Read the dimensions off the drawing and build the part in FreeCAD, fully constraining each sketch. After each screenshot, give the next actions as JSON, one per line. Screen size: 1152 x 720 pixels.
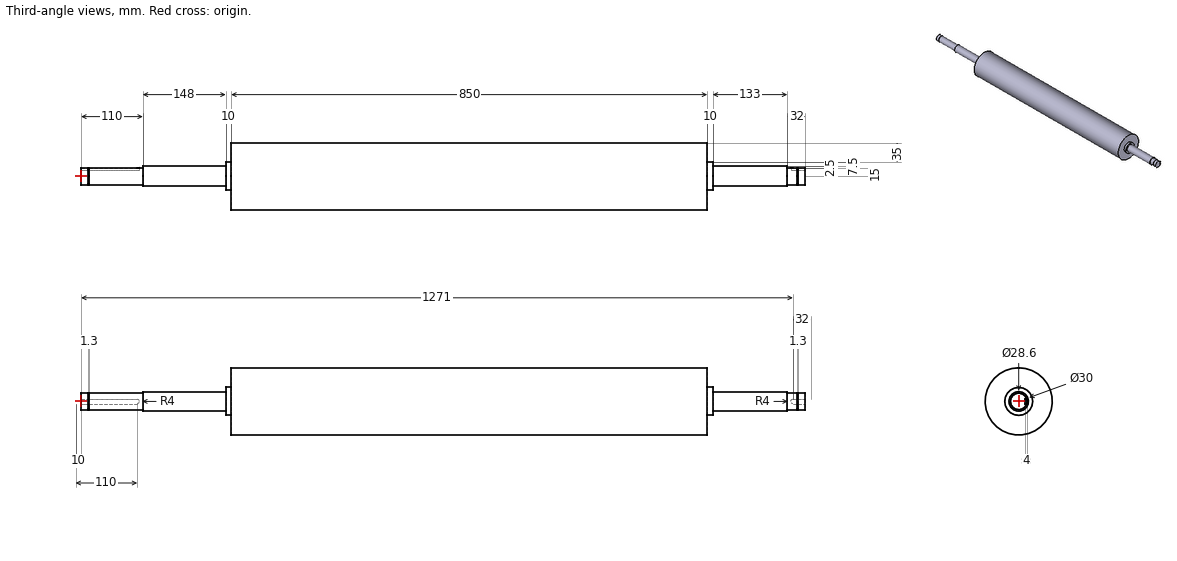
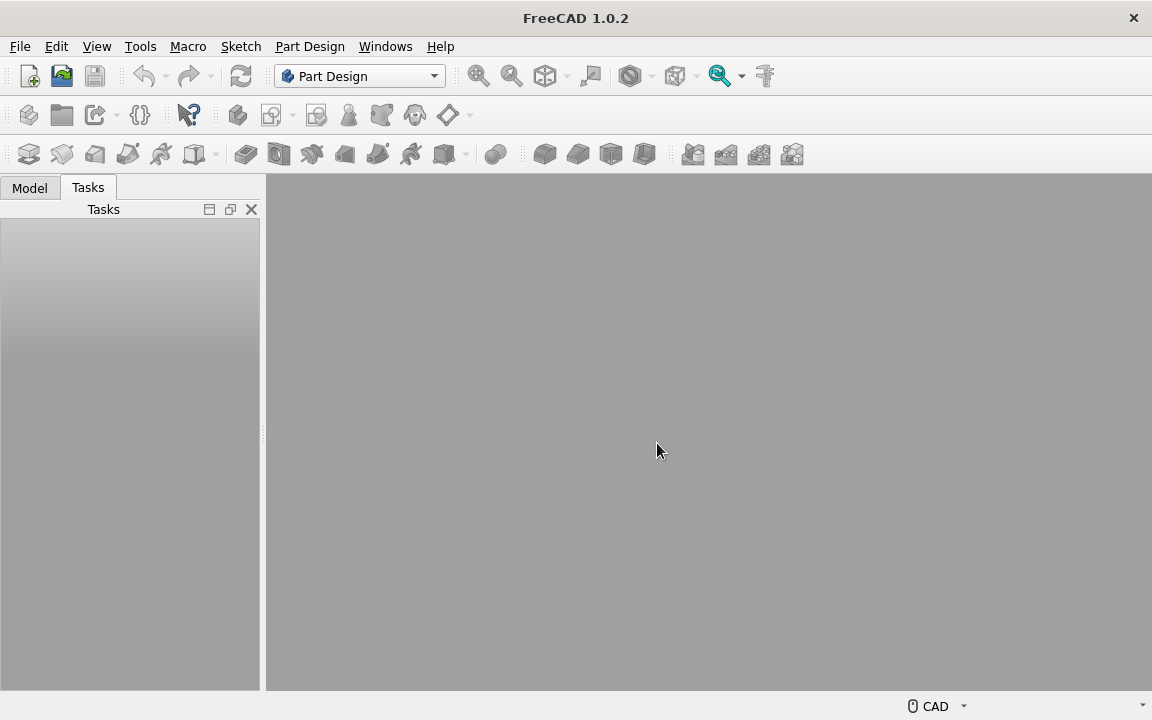
{"action": "key", "text": "ctrl+n"}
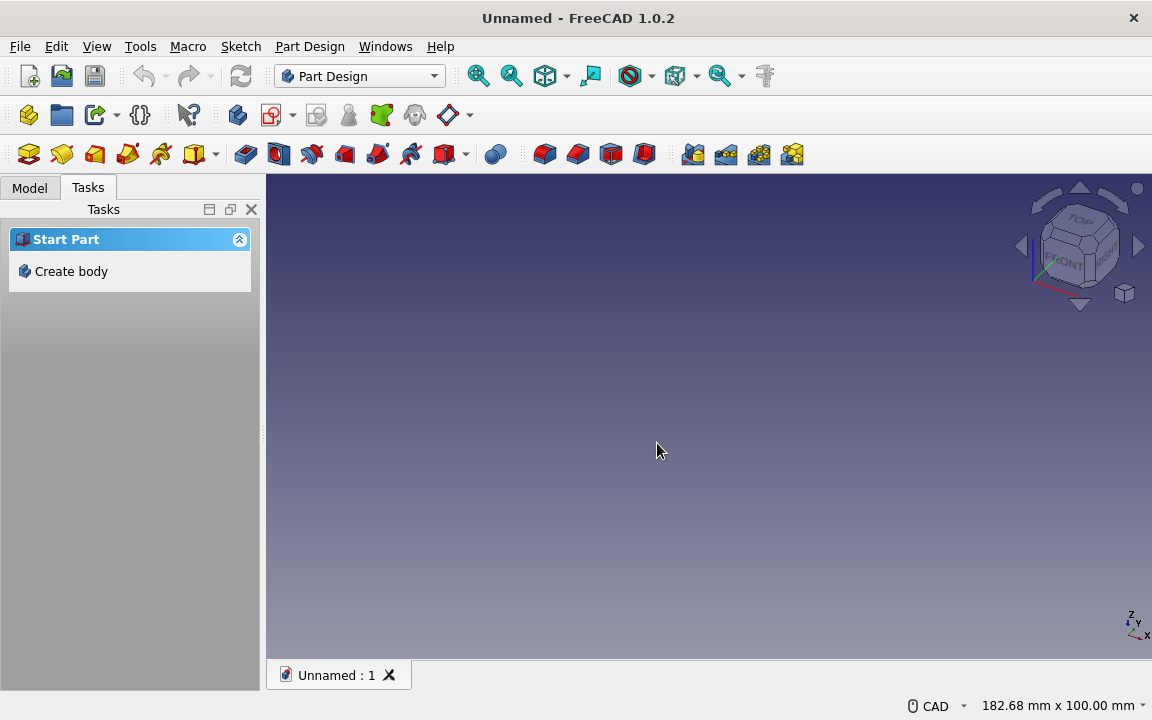
{"action": "left_click", "coordinate": [270, 116]}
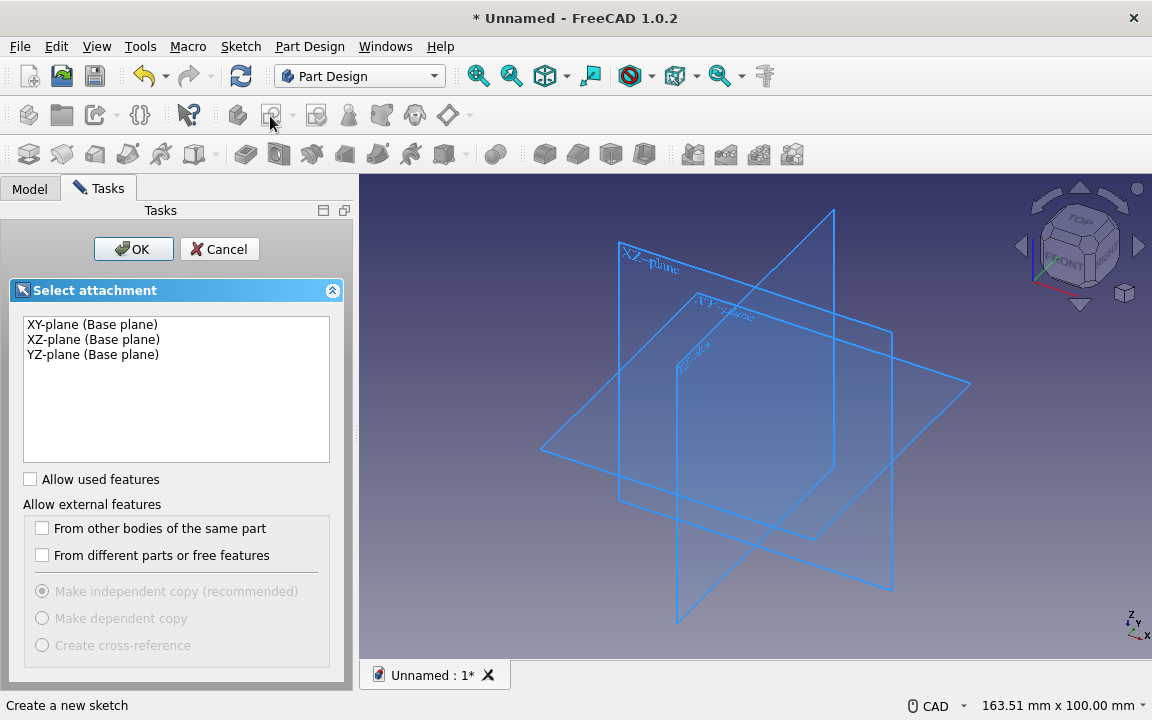
{"action": "left_click", "coordinate": [84, 324]}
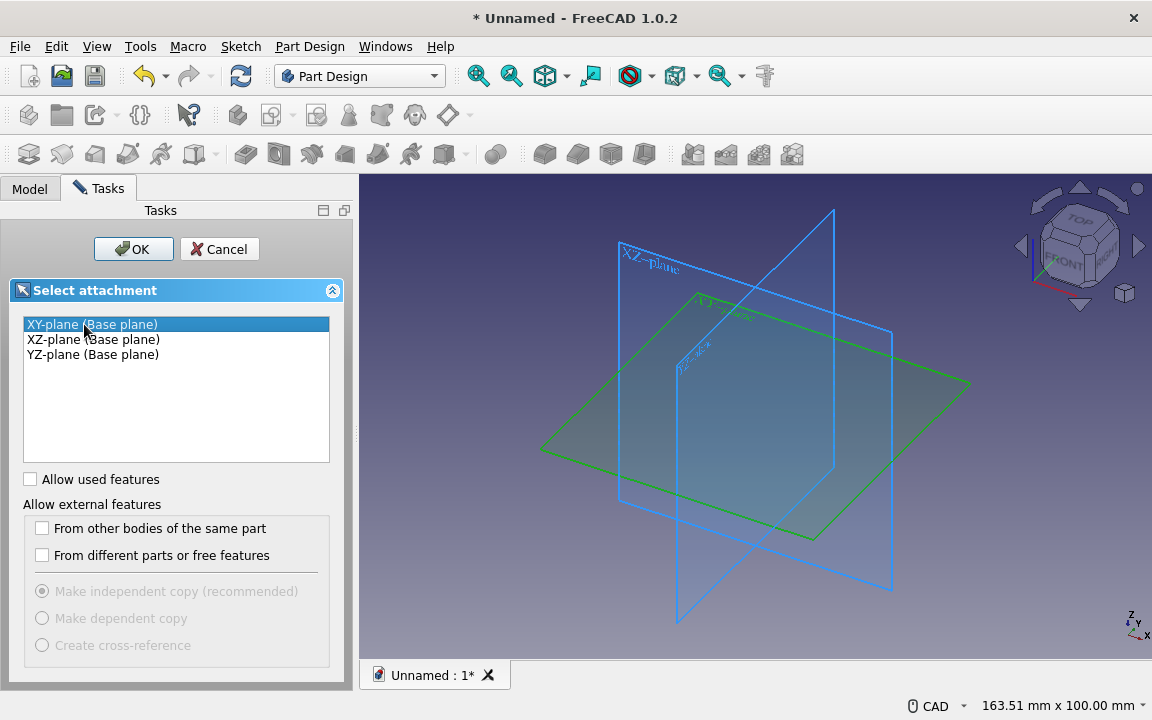
{"action": "left_click", "coordinate": [134, 249]}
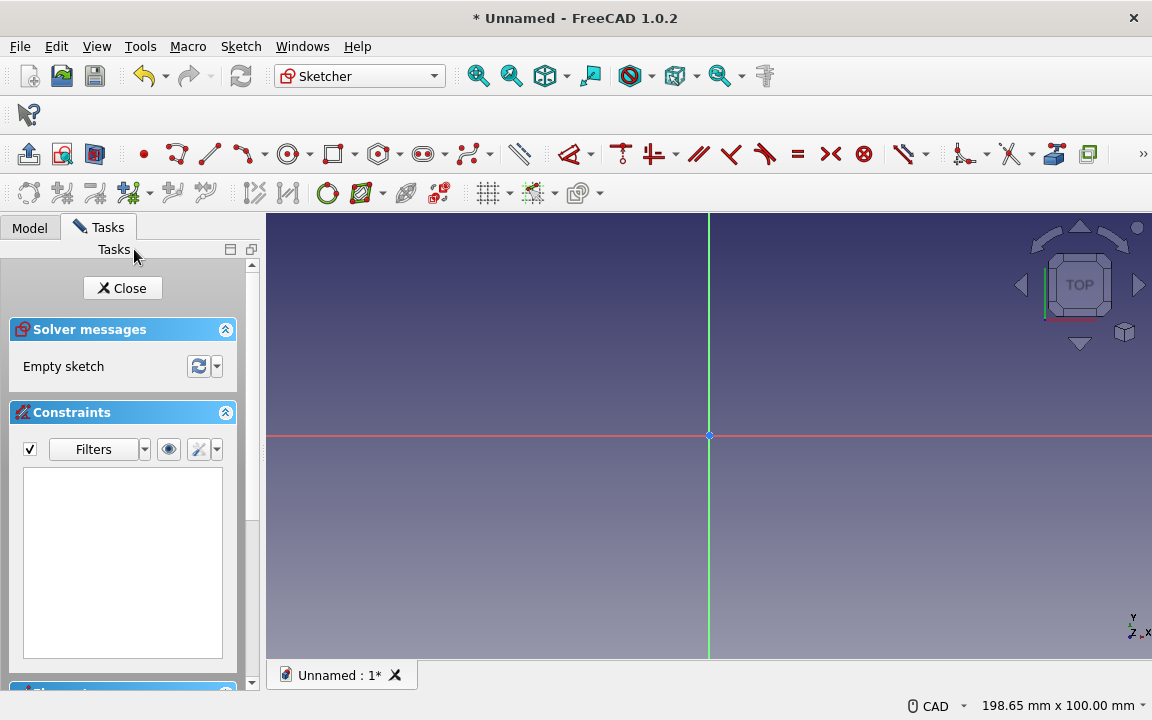
{"action": "scroll", "coordinate": [346, 449], "scroll_direction": "down", "scroll_amount": 12}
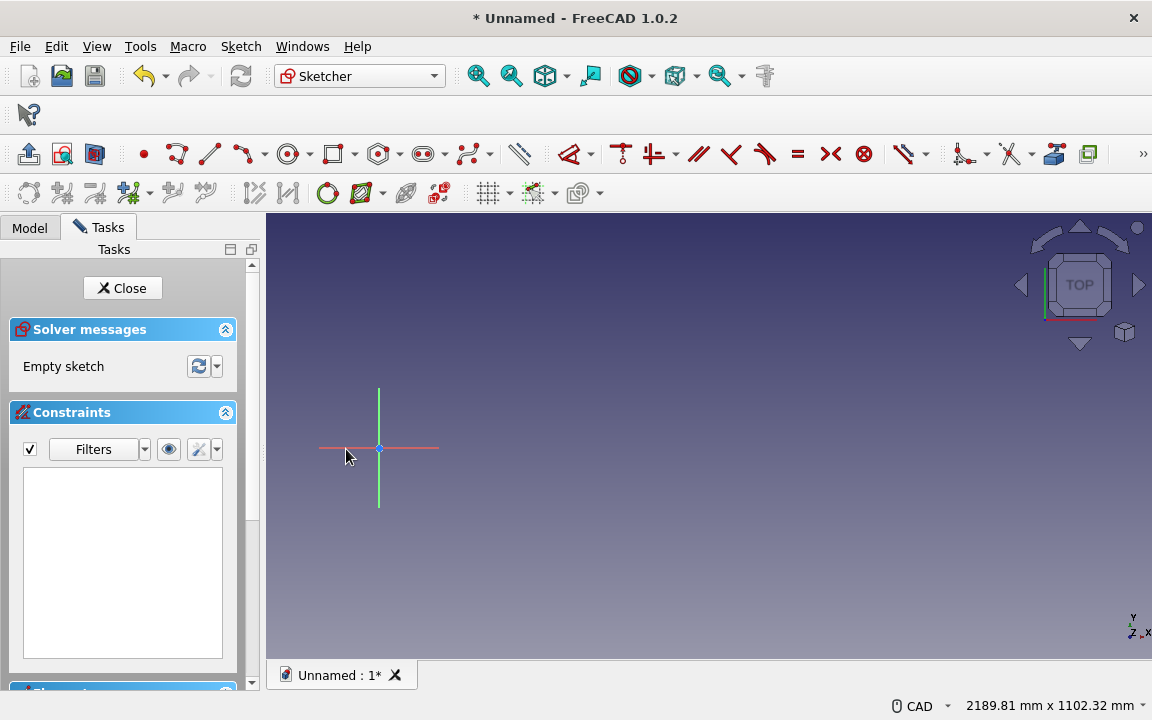
{"action": "left_click", "coordinate": [177, 154]}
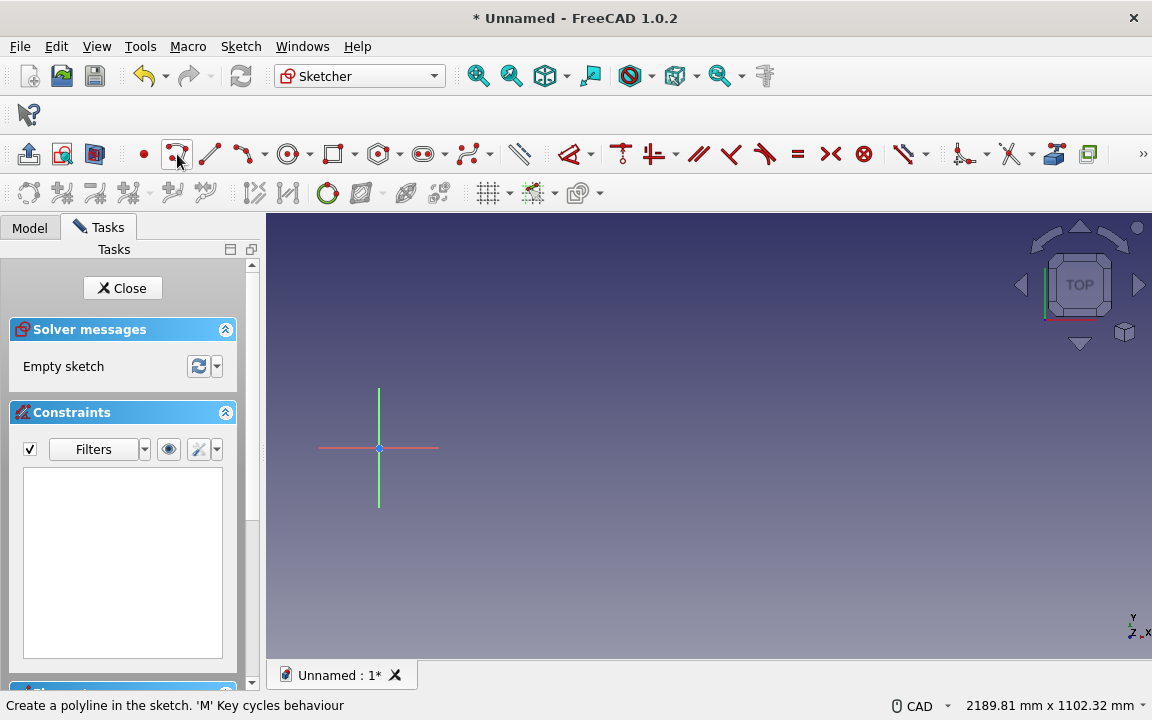
{"action": "left_click", "coordinate": [379, 448]}
{"action": "left_click", "coordinate": [902, 439]}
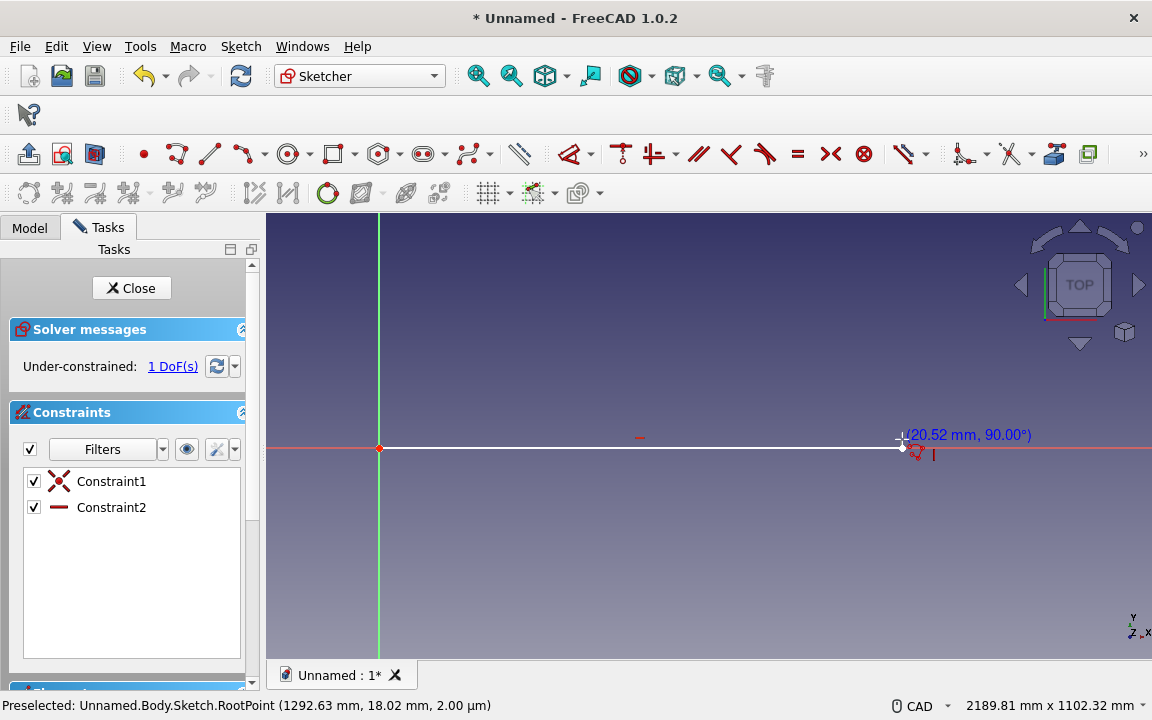
{"action": "scroll", "coordinate": [902, 442], "scroll_direction": "up", "scroll_amount": 5}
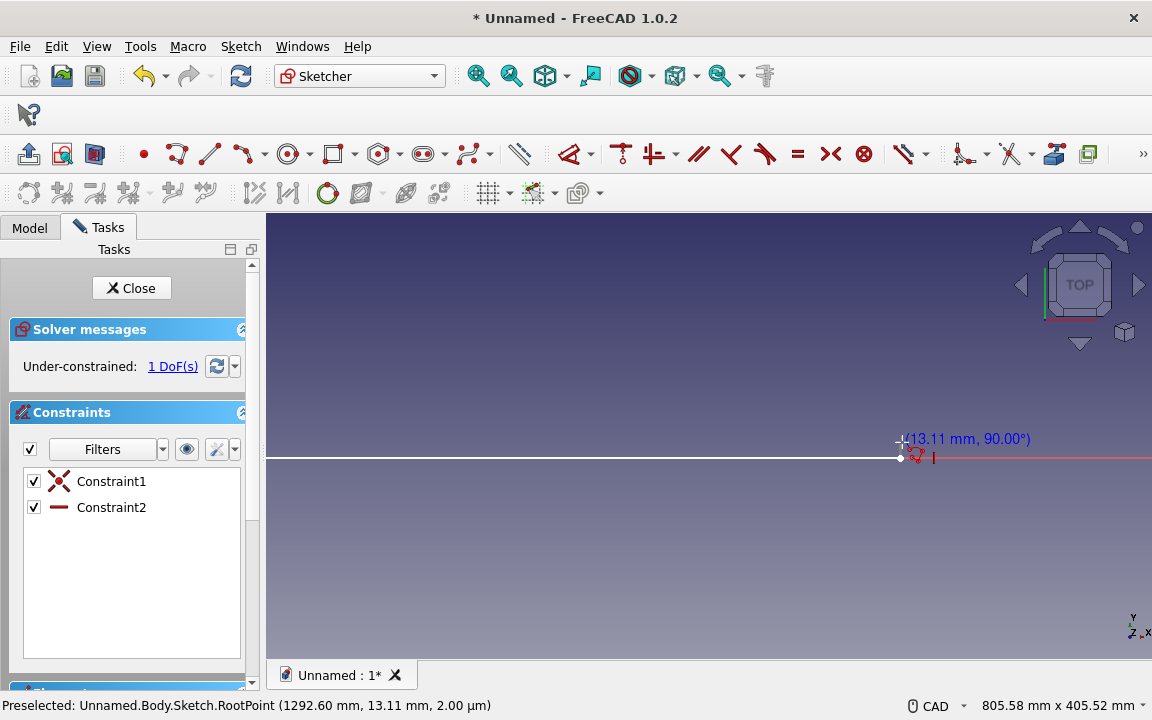
{"action": "left_click", "coordinate": [901, 442]}
{"action": "left_click", "coordinate": [866, 442]}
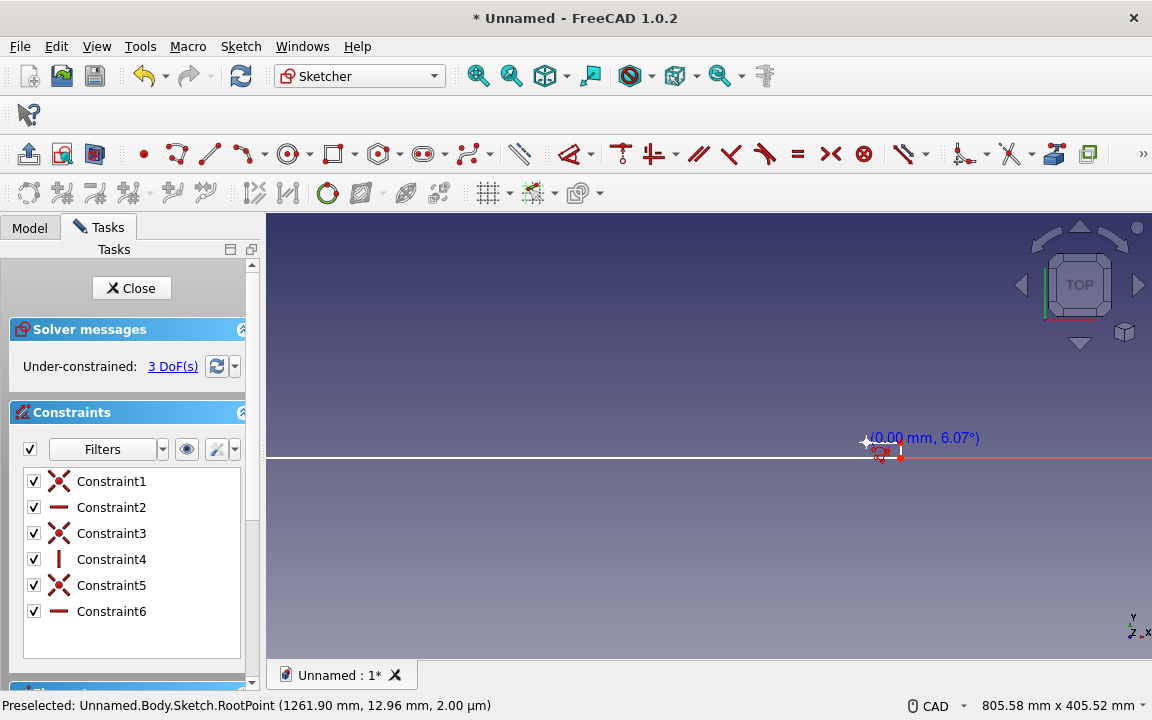
{"action": "scroll", "coordinate": [866, 439], "scroll_direction": "up", "scroll_amount": 9}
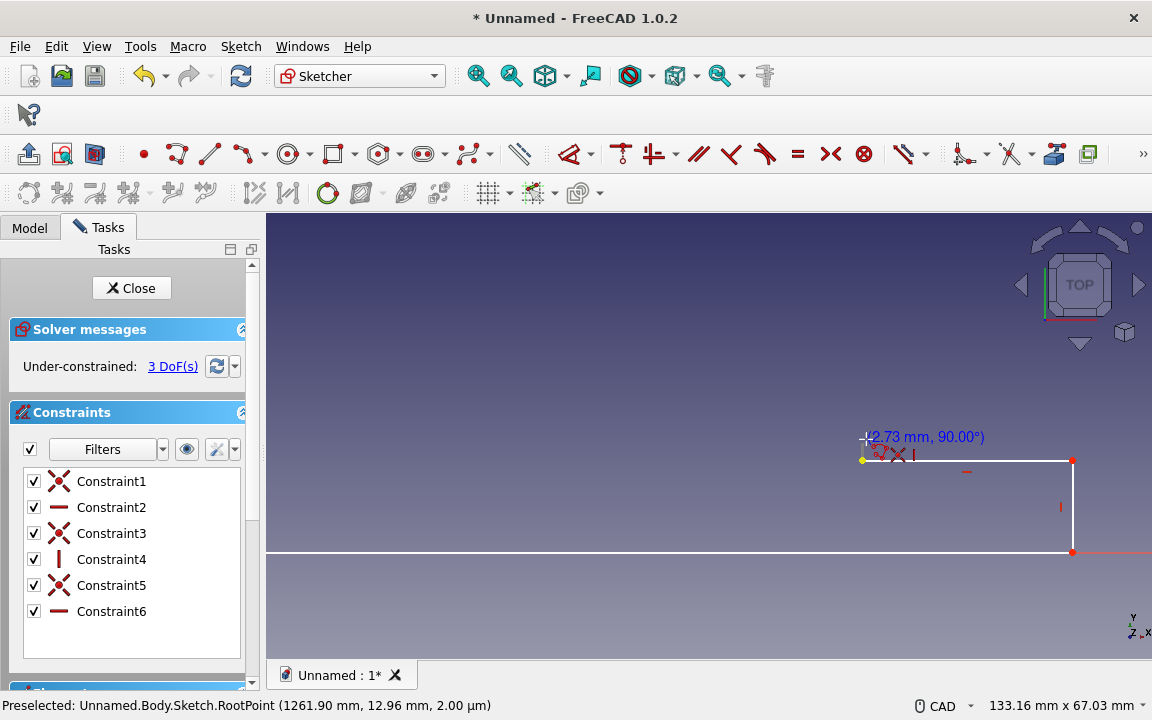
{"action": "left_click", "coordinate": [863, 436]}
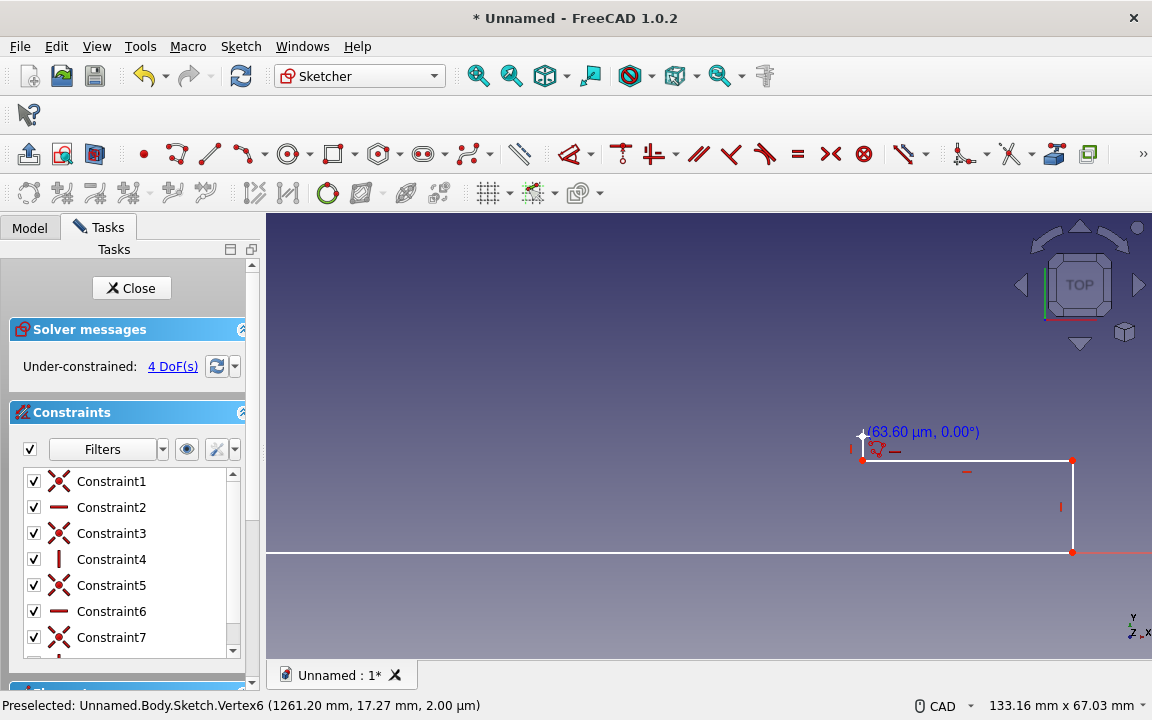
{"action": "scroll", "coordinate": [891, 441], "scroll_direction": "down", "scroll_amount": 14}